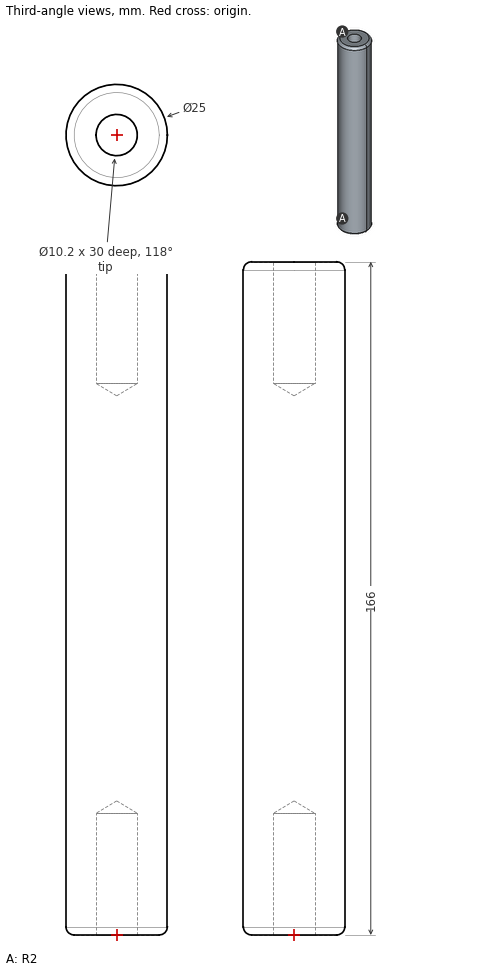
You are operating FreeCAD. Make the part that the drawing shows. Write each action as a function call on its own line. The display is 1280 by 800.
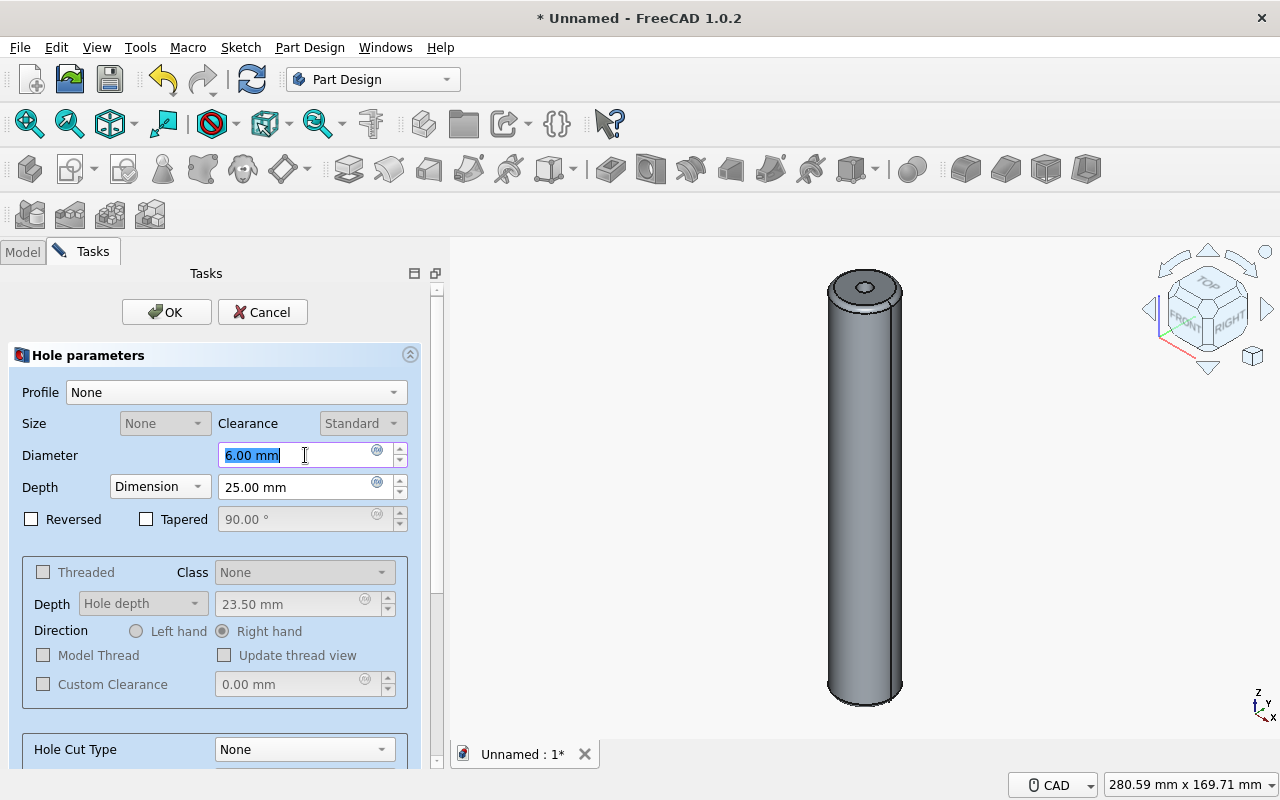
text(10.2)
key(Tab)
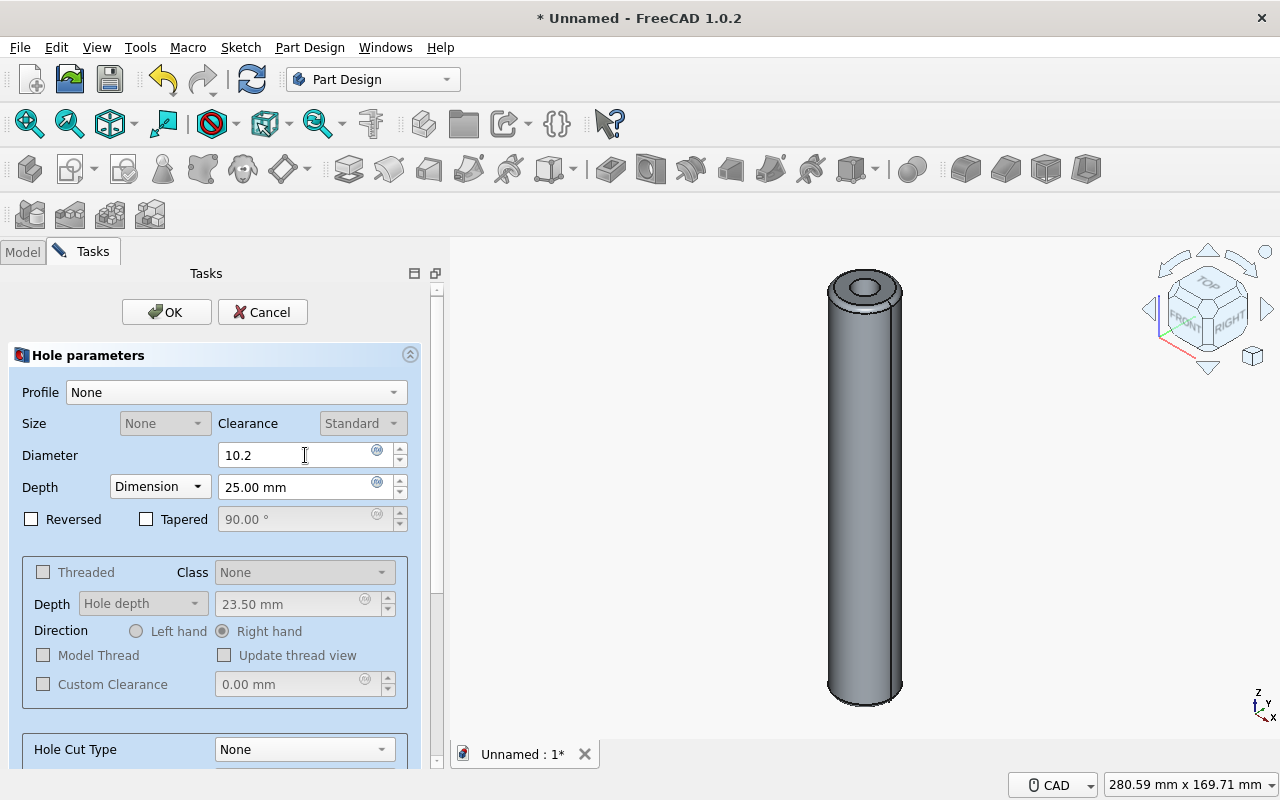
triple_click(305, 487)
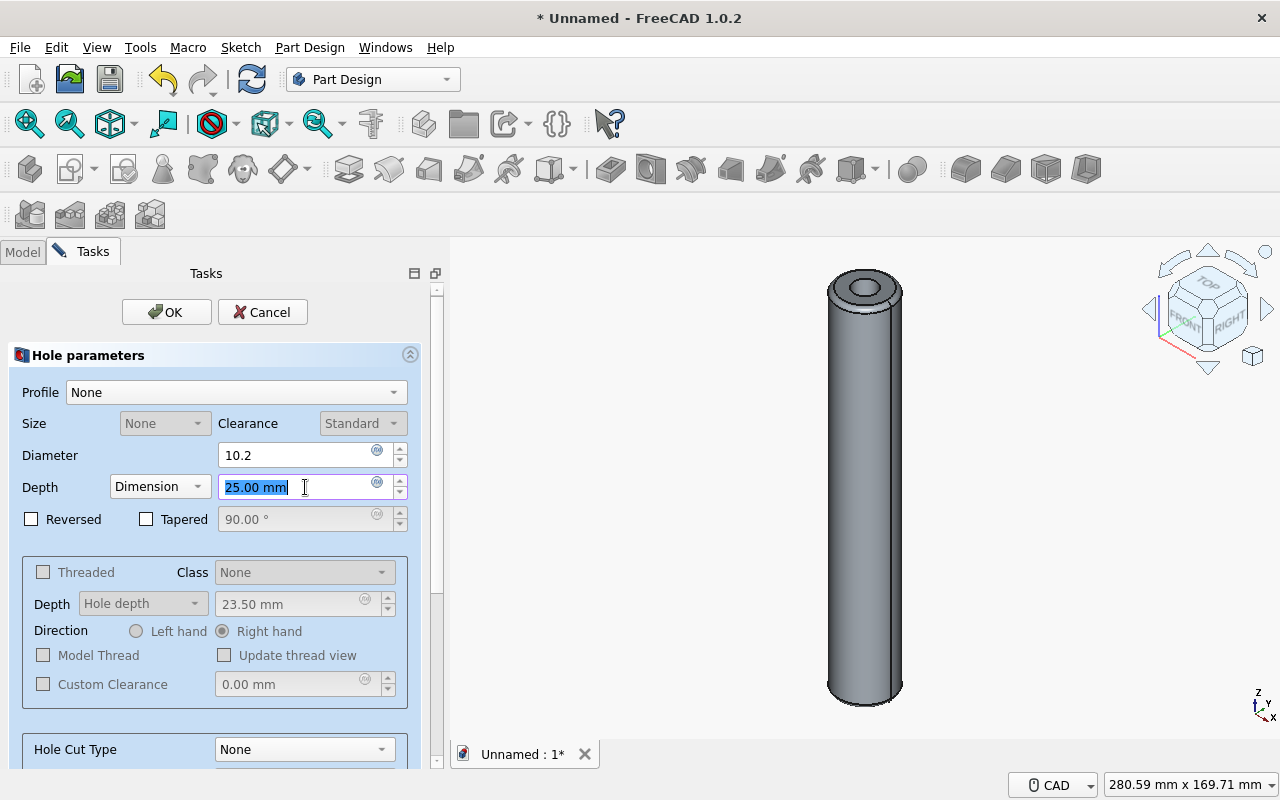
text(30)
key(Tab)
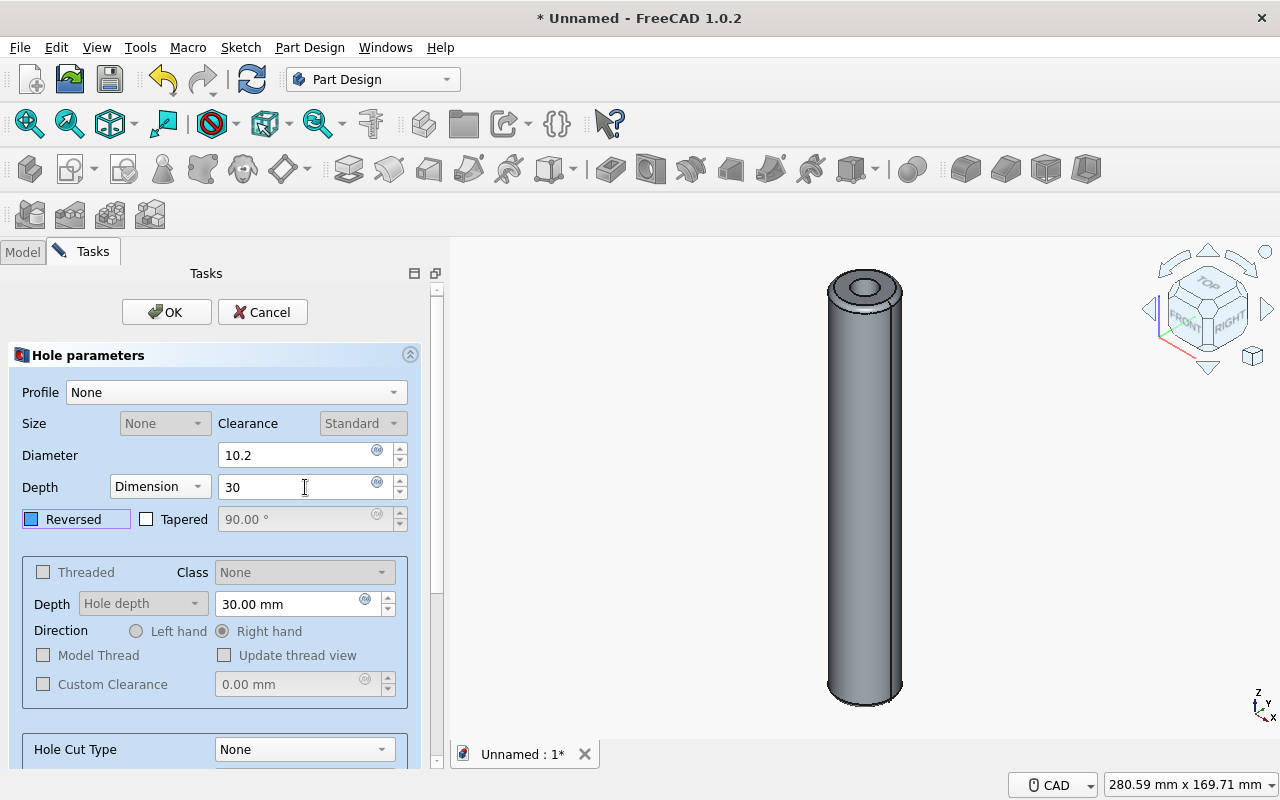
click(167, 312)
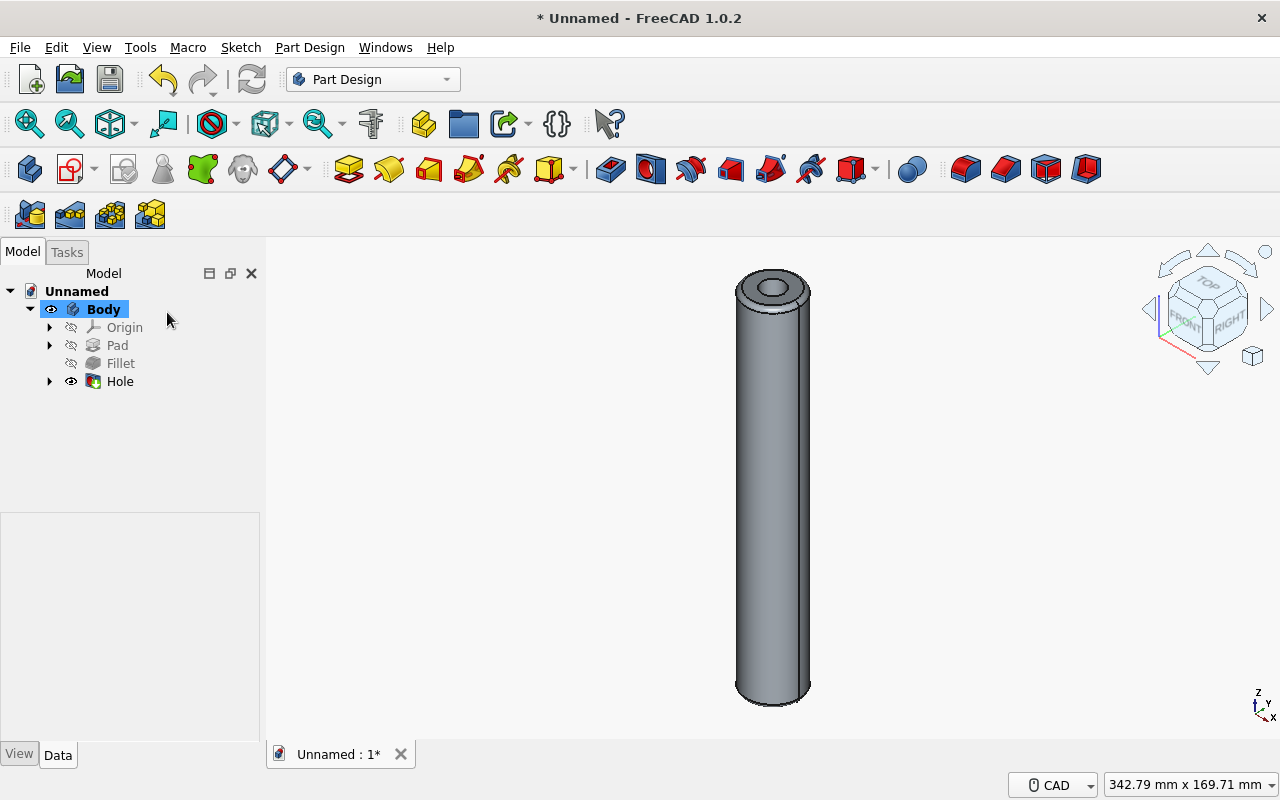
click(70, 170)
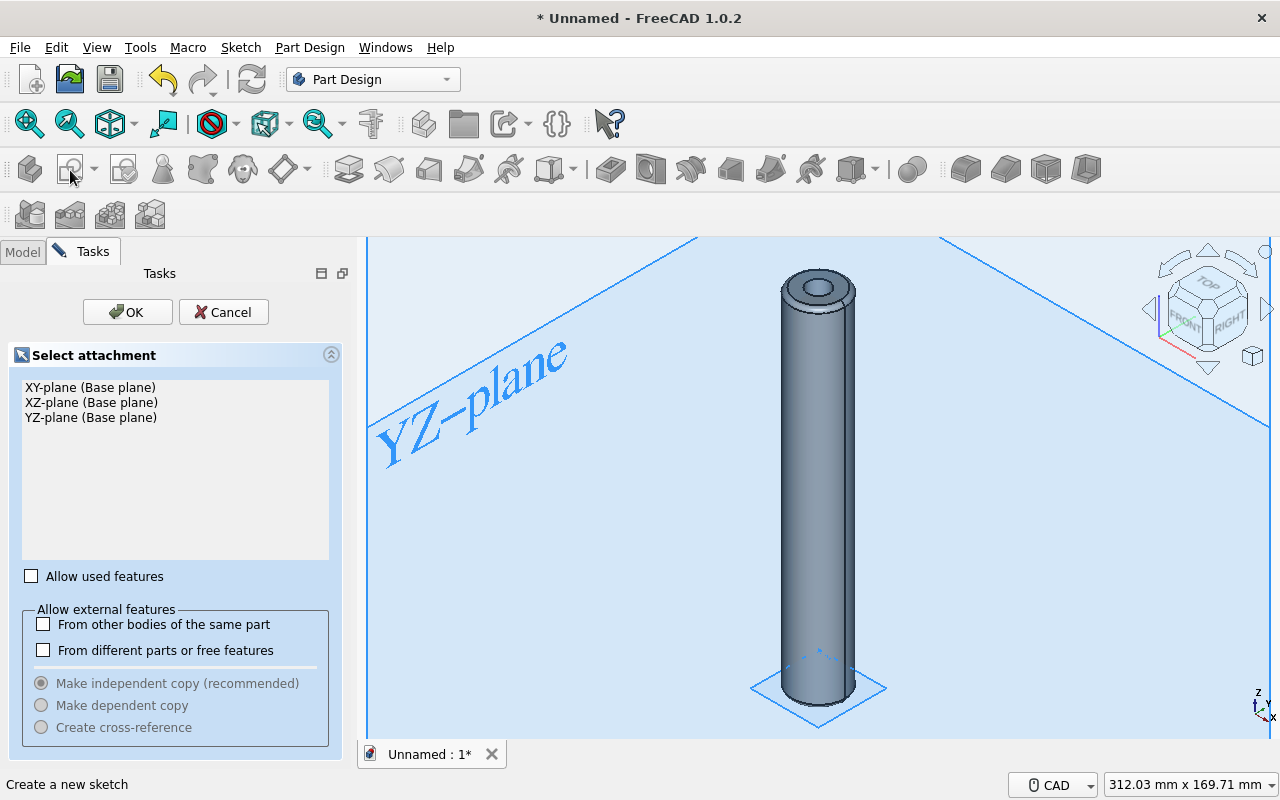
click(82, 388)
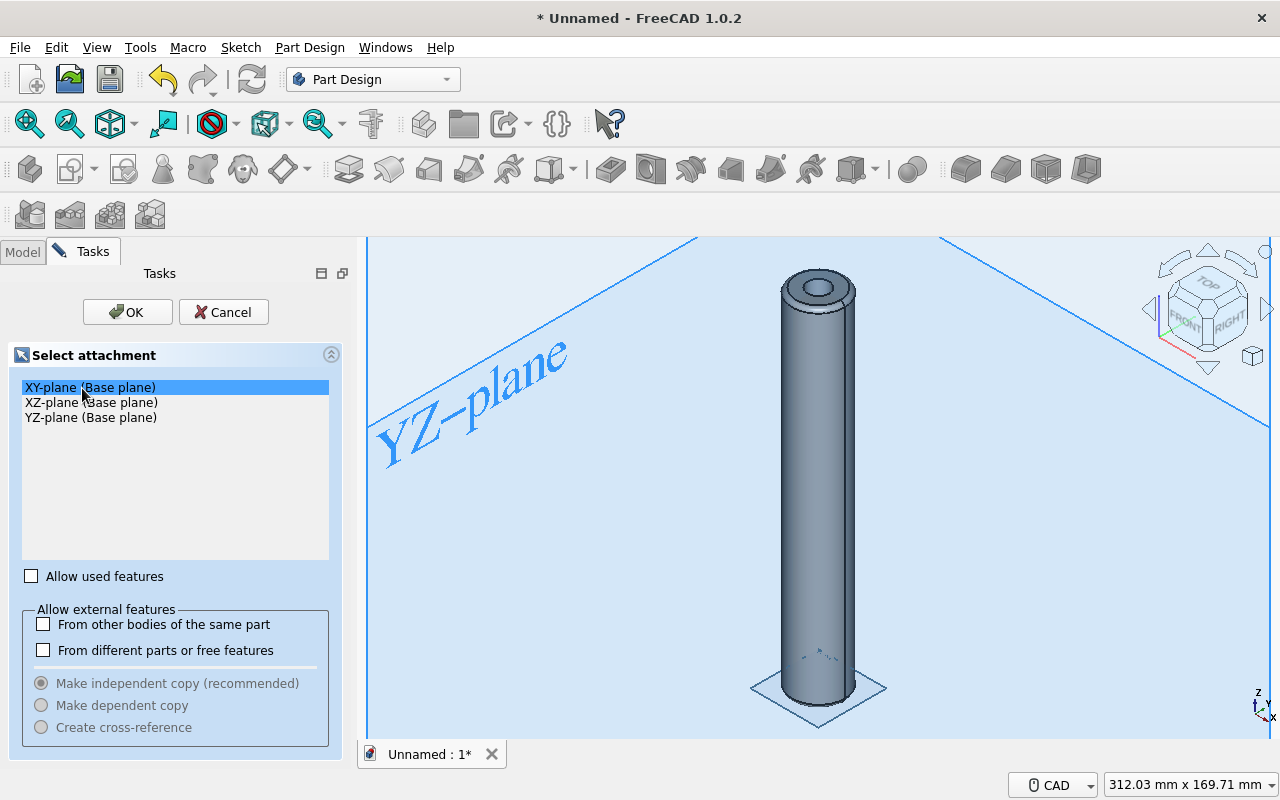
click(128, 312)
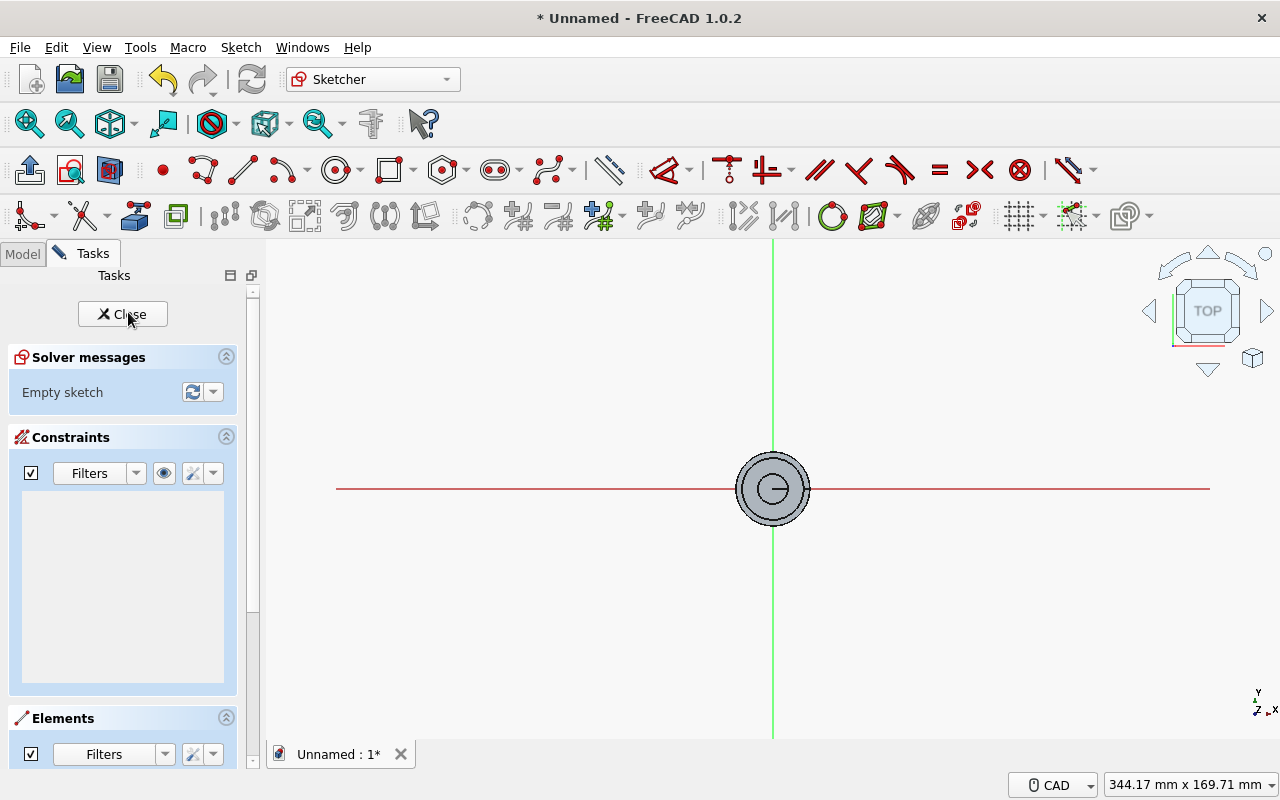
click(110, 170)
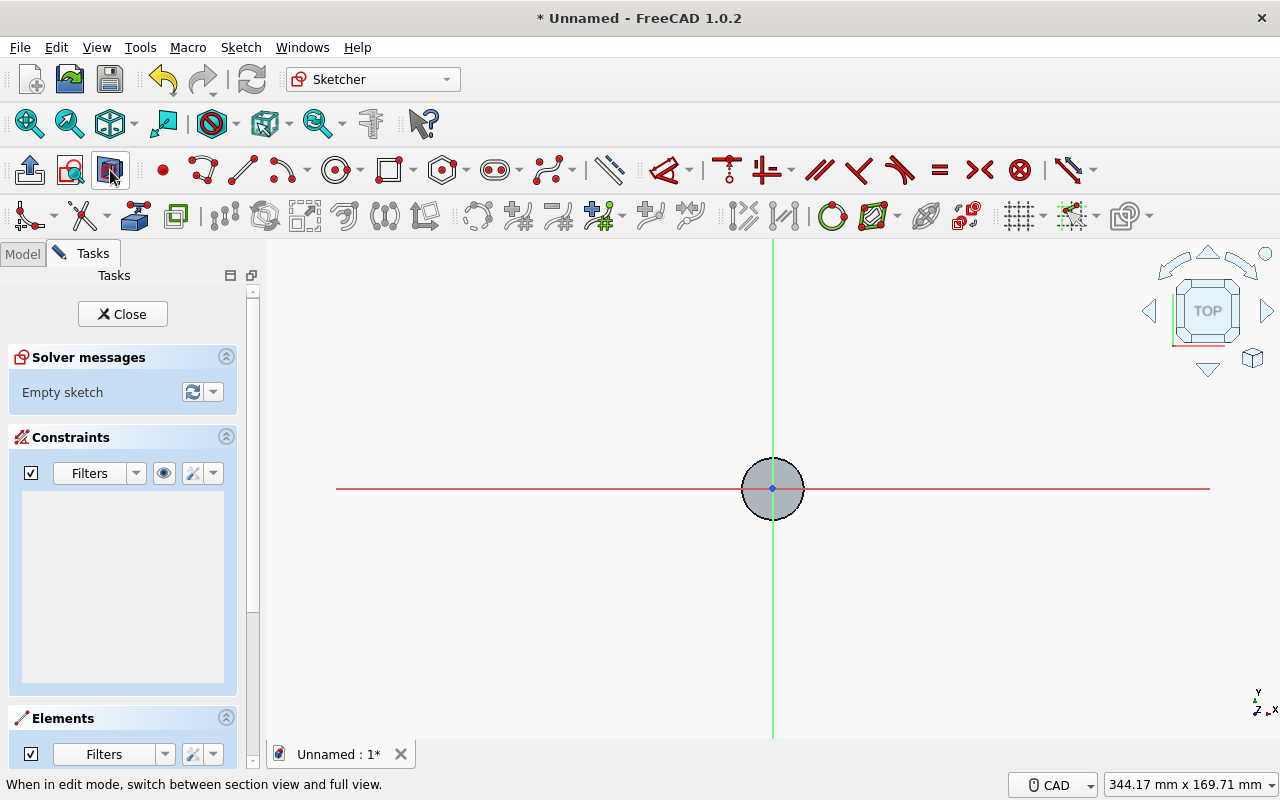
scroll(780, 489, up, 12)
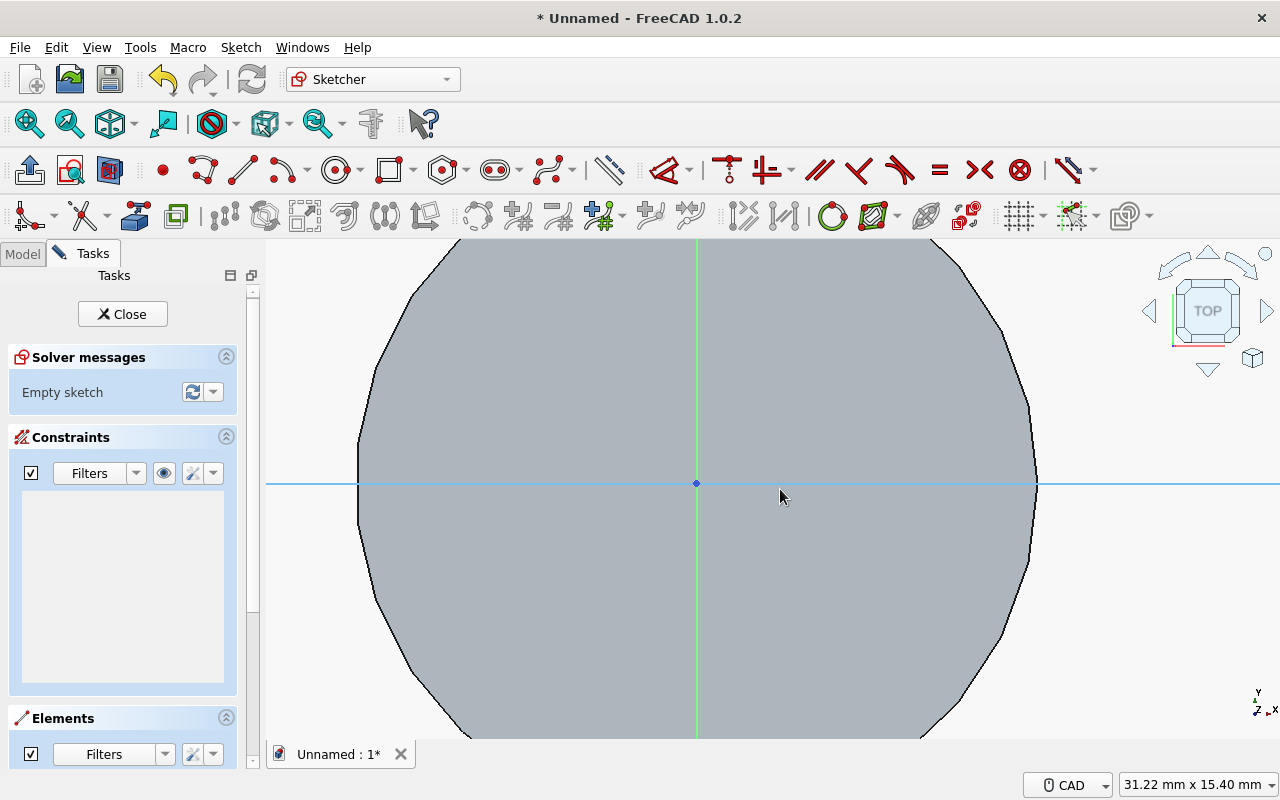
click(336, 170)